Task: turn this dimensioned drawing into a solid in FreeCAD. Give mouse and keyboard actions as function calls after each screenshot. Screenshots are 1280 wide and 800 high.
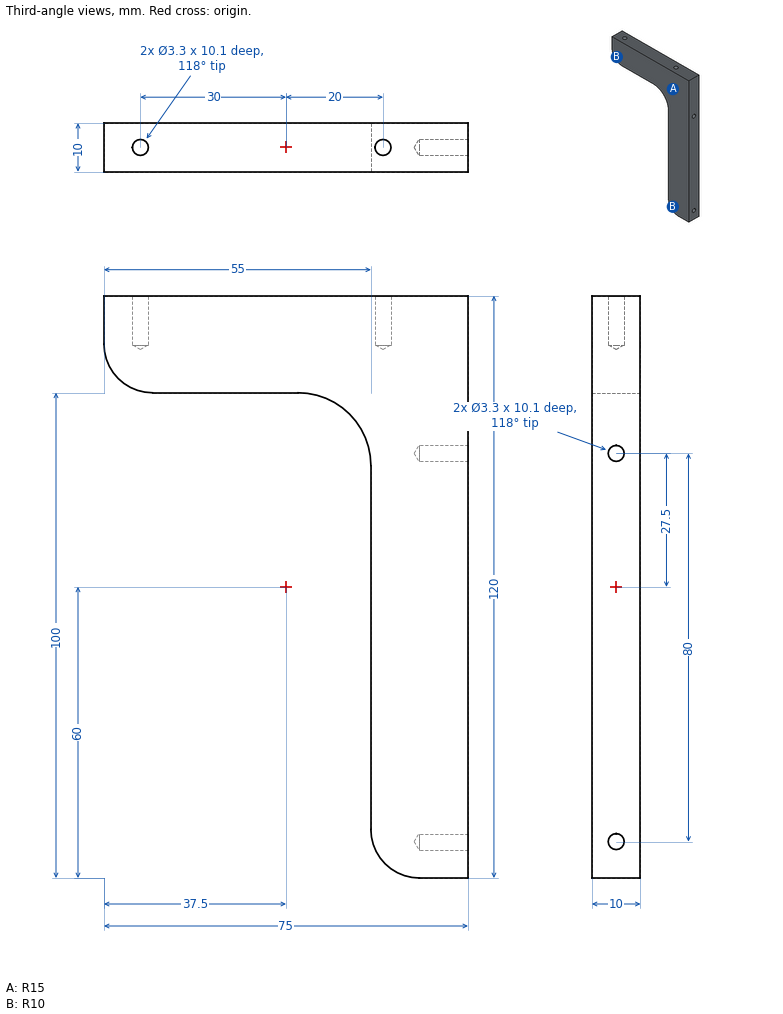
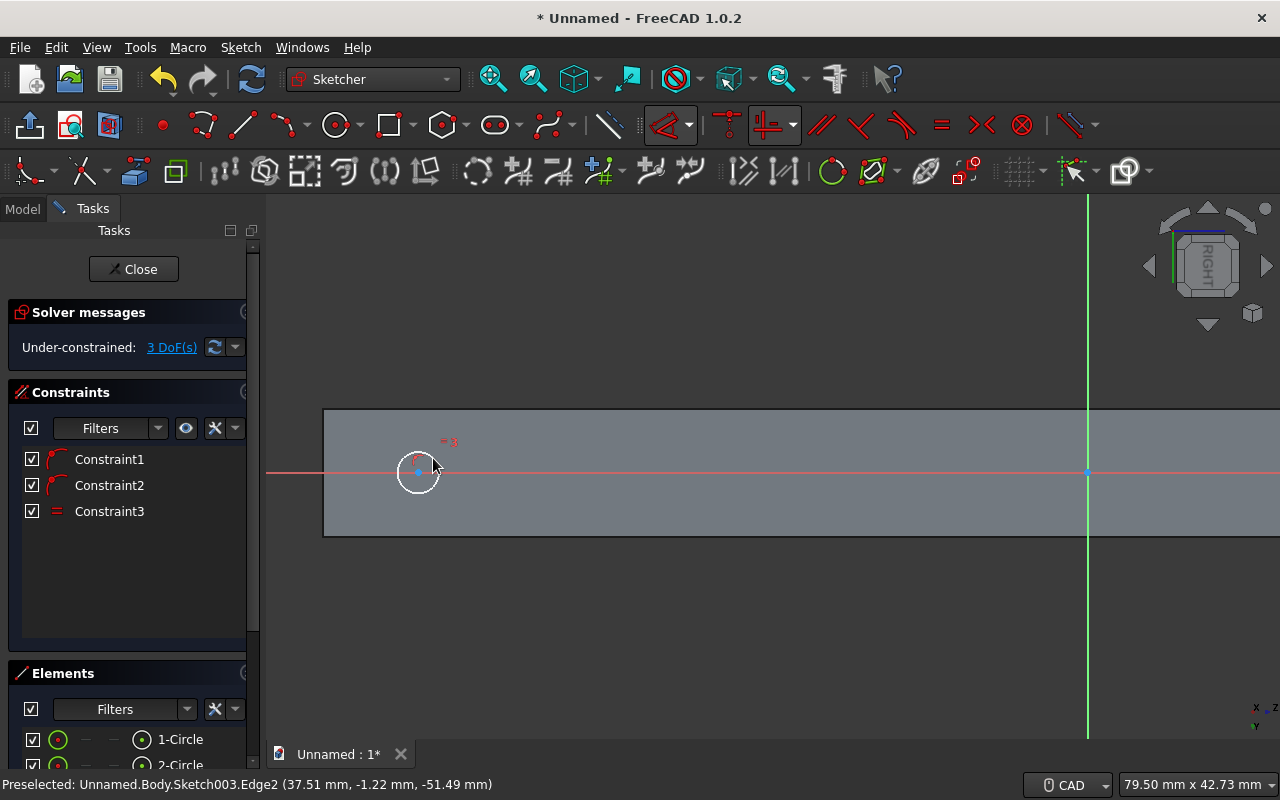
click(664, 126)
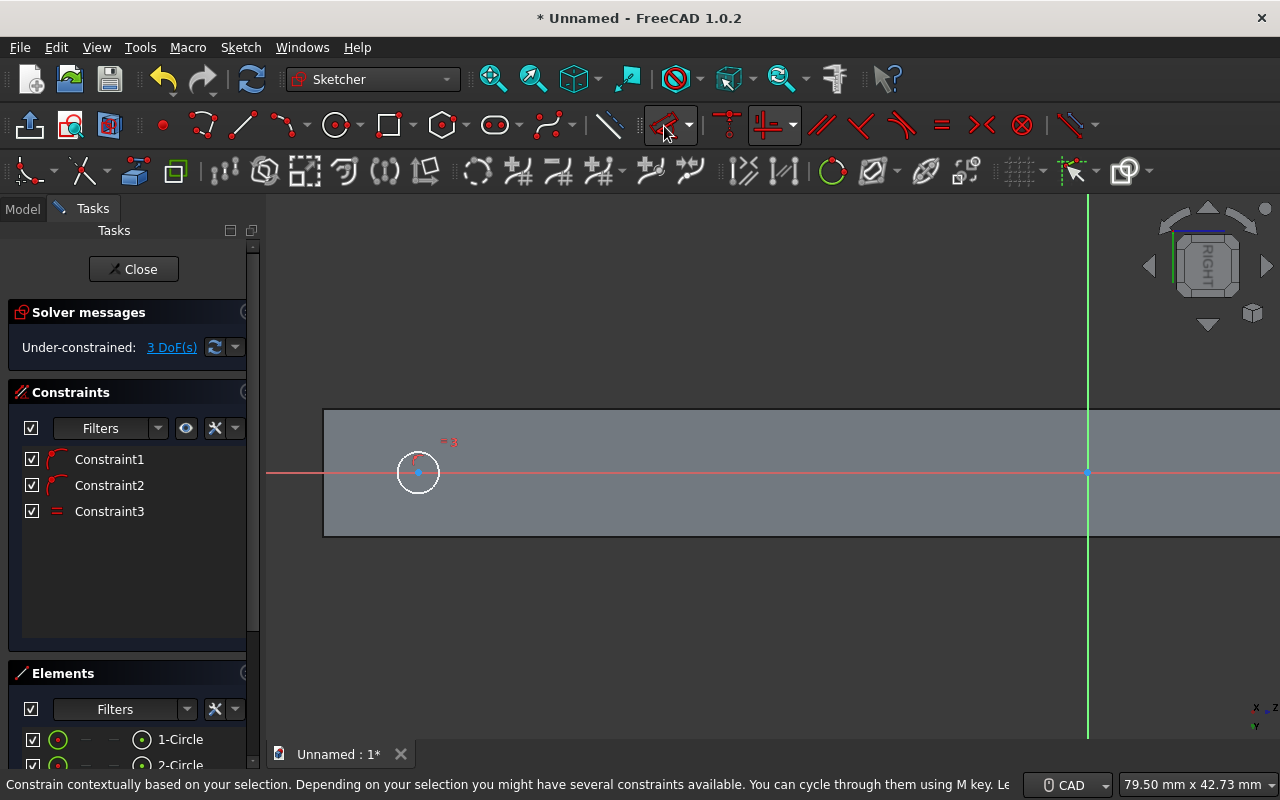
scroll(432, 459, down, 3)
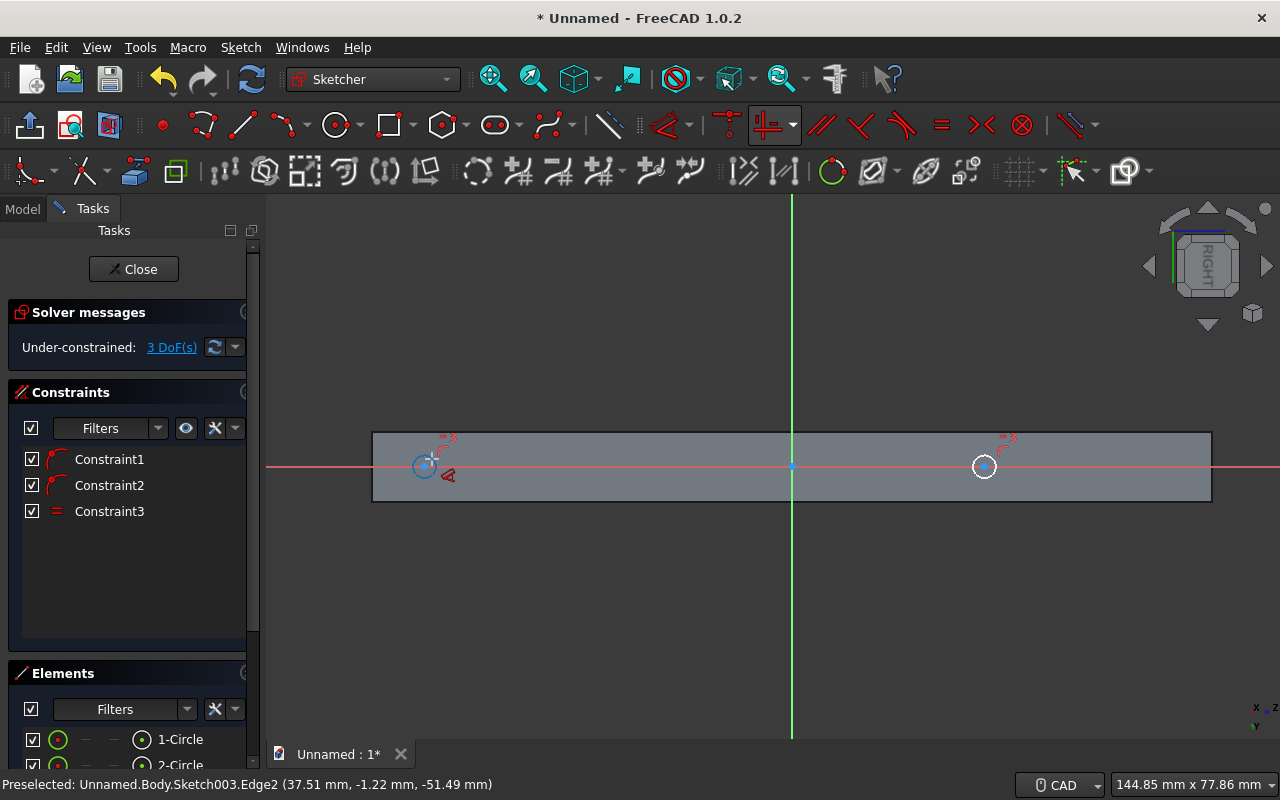
scroll(992, 459, up, 3)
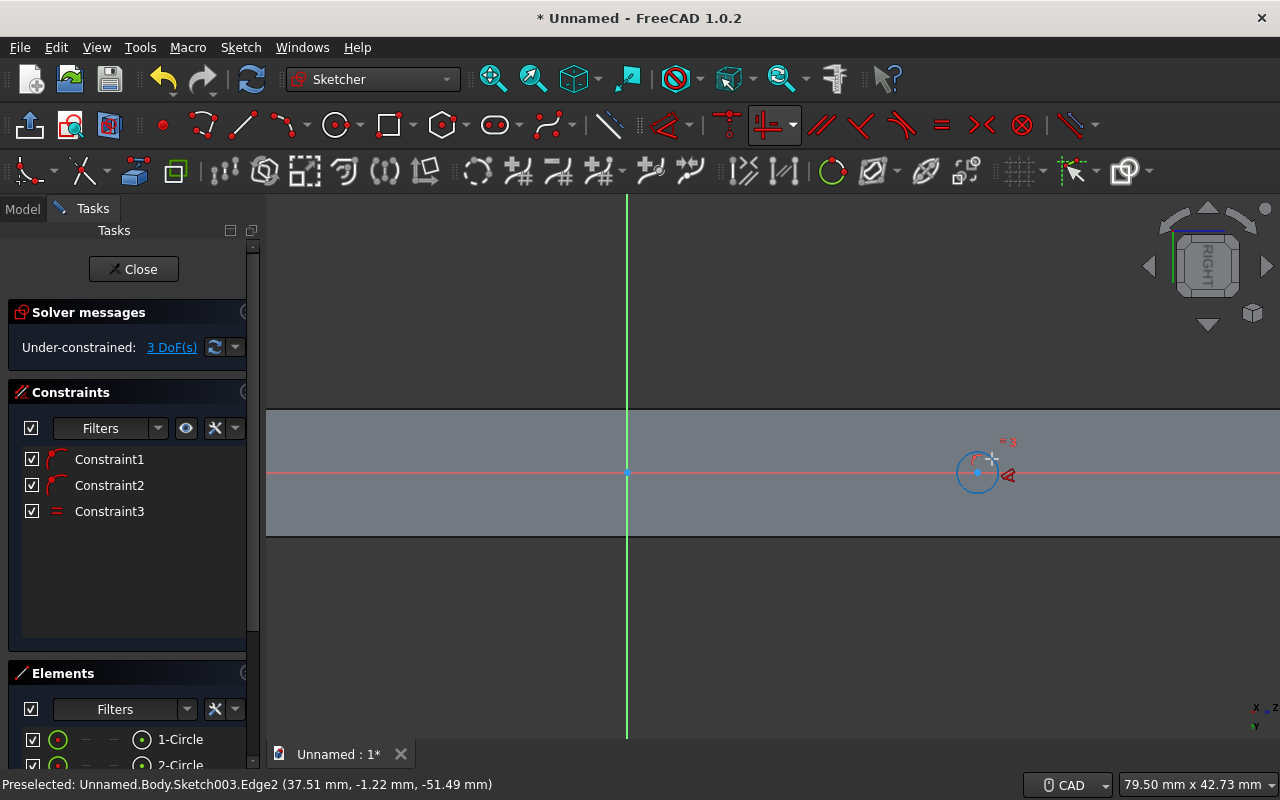
click(992, 458)
click(1014, 435)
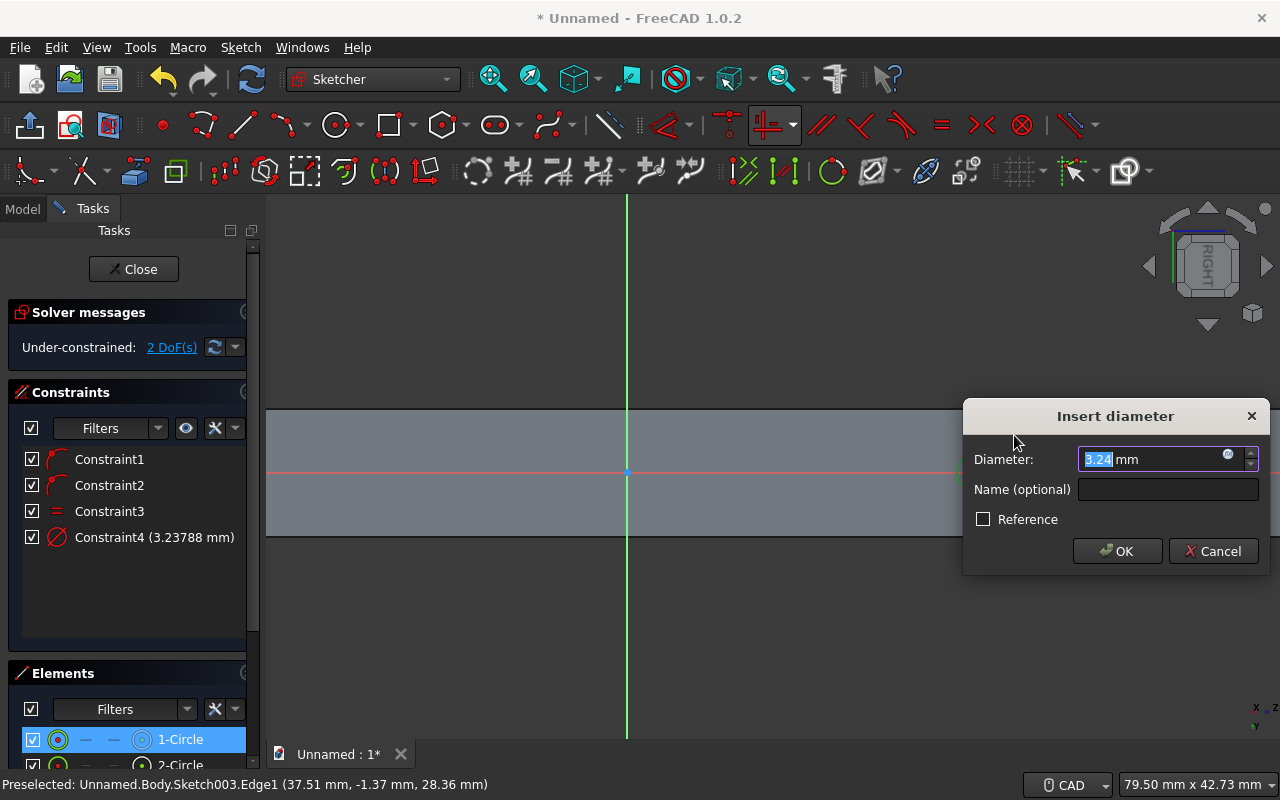
text(3.3)
key(Return)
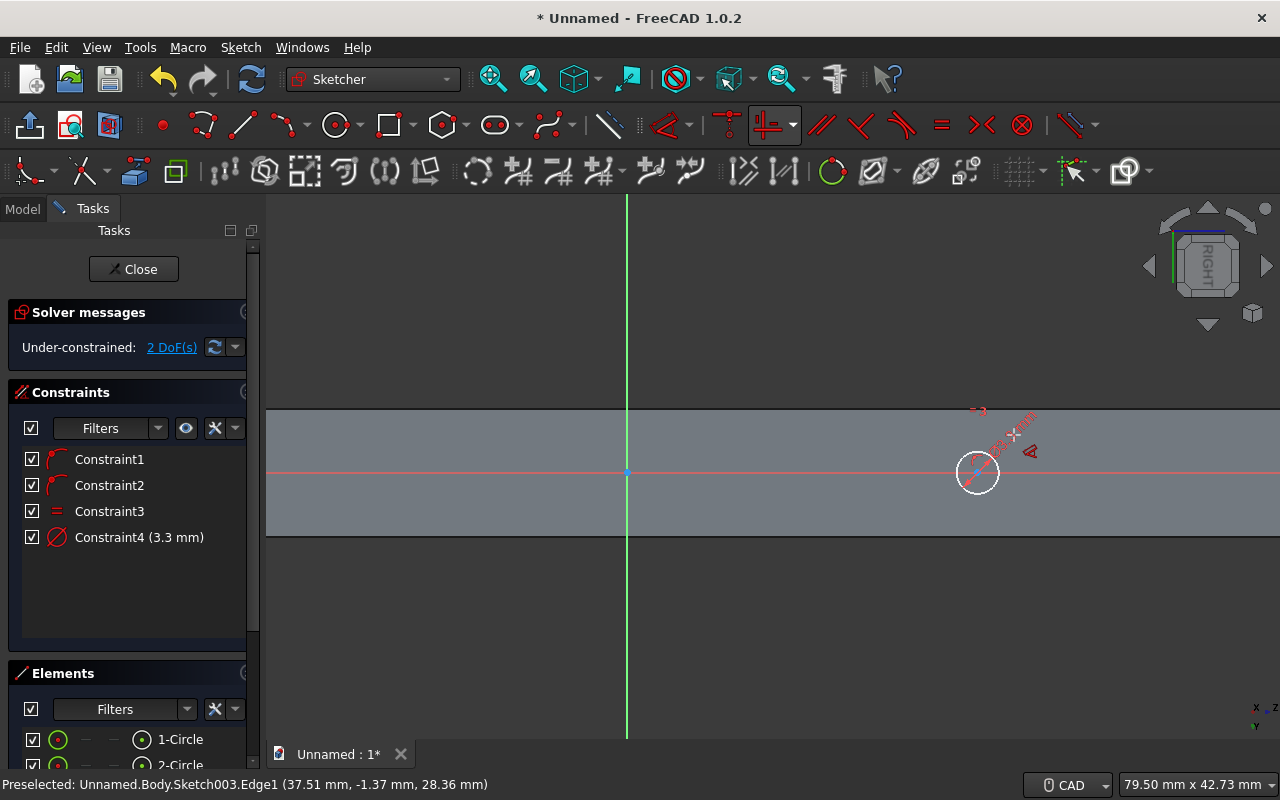
click(978, 473)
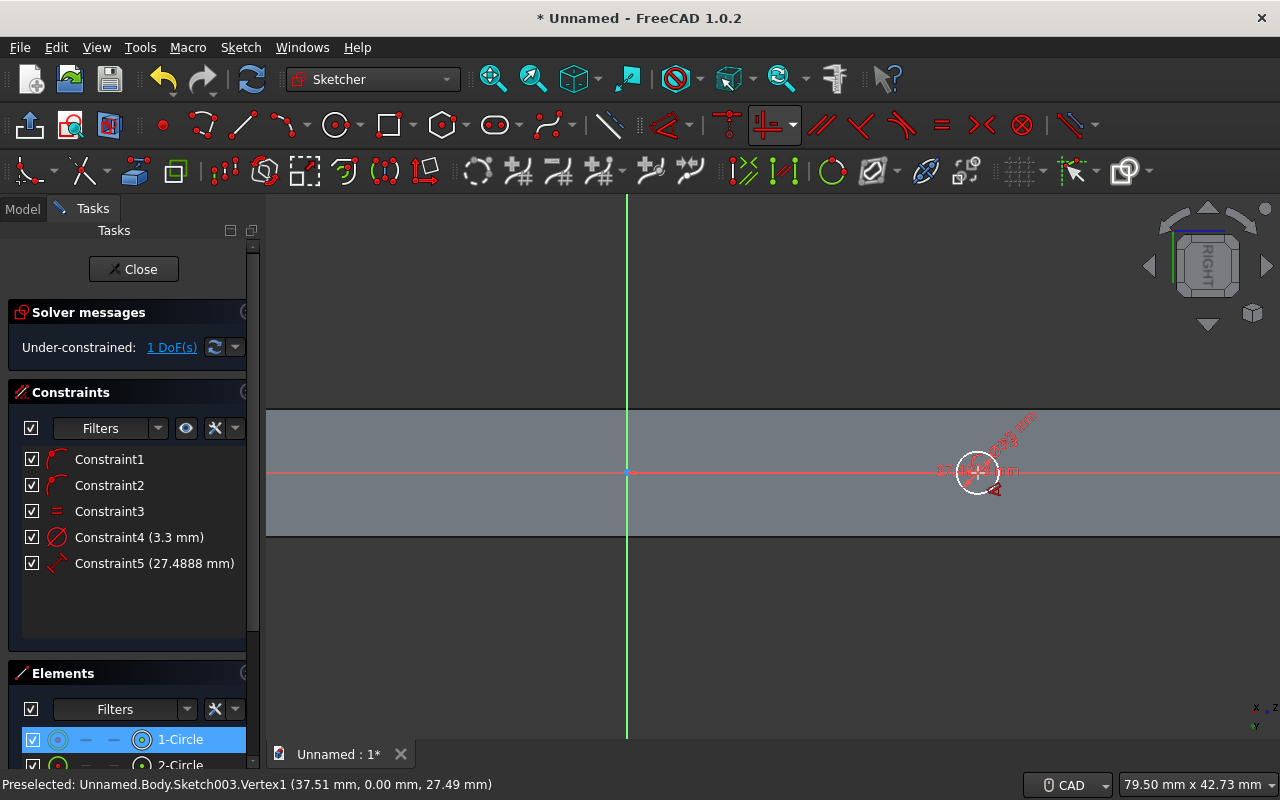
scroll(993, 459, down, 3)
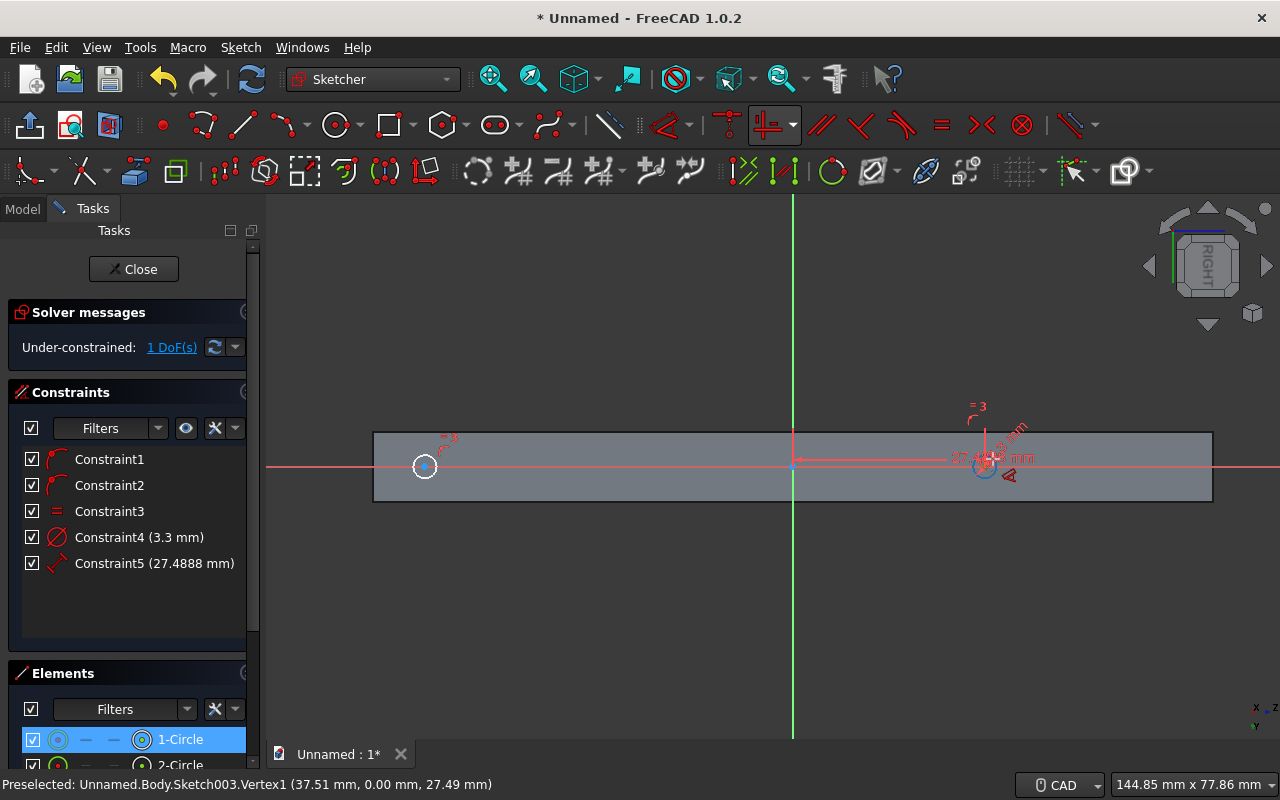
click(425, 467)
click(705, 501)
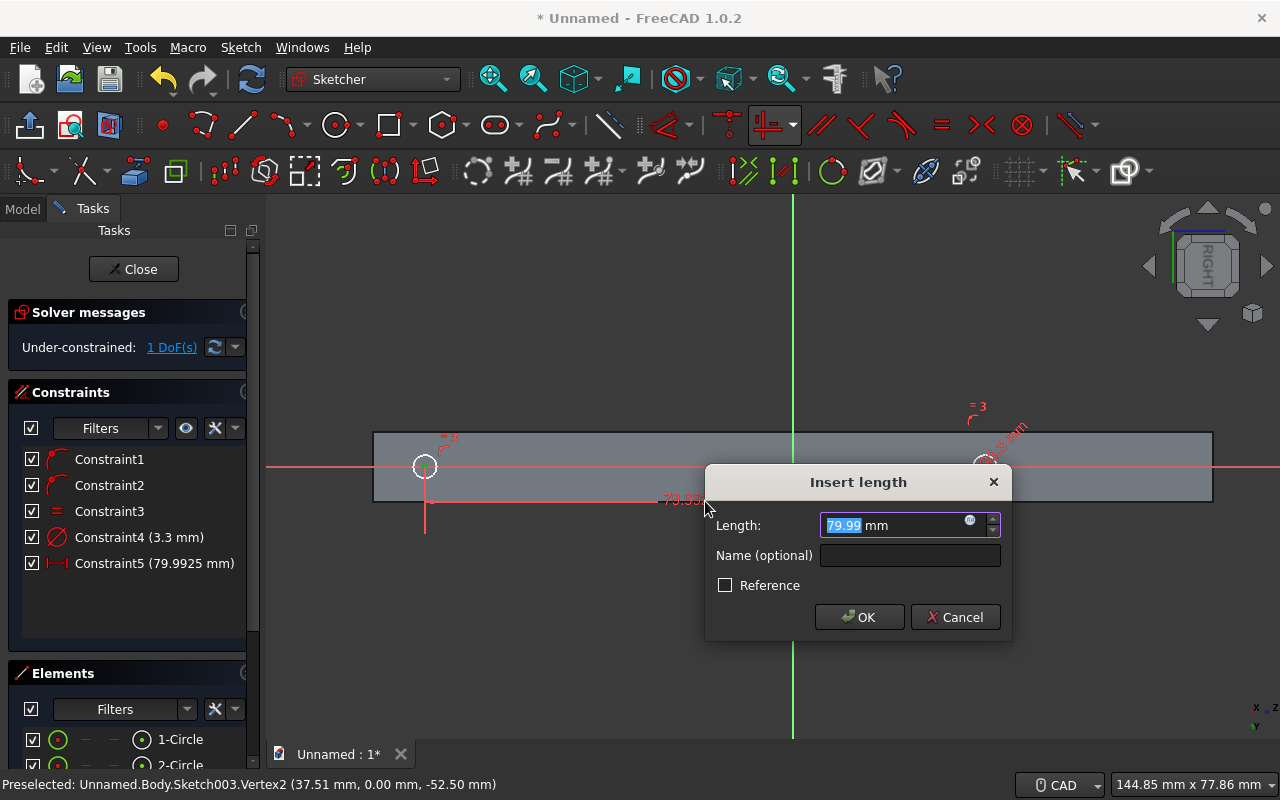
text(80)
key(Return)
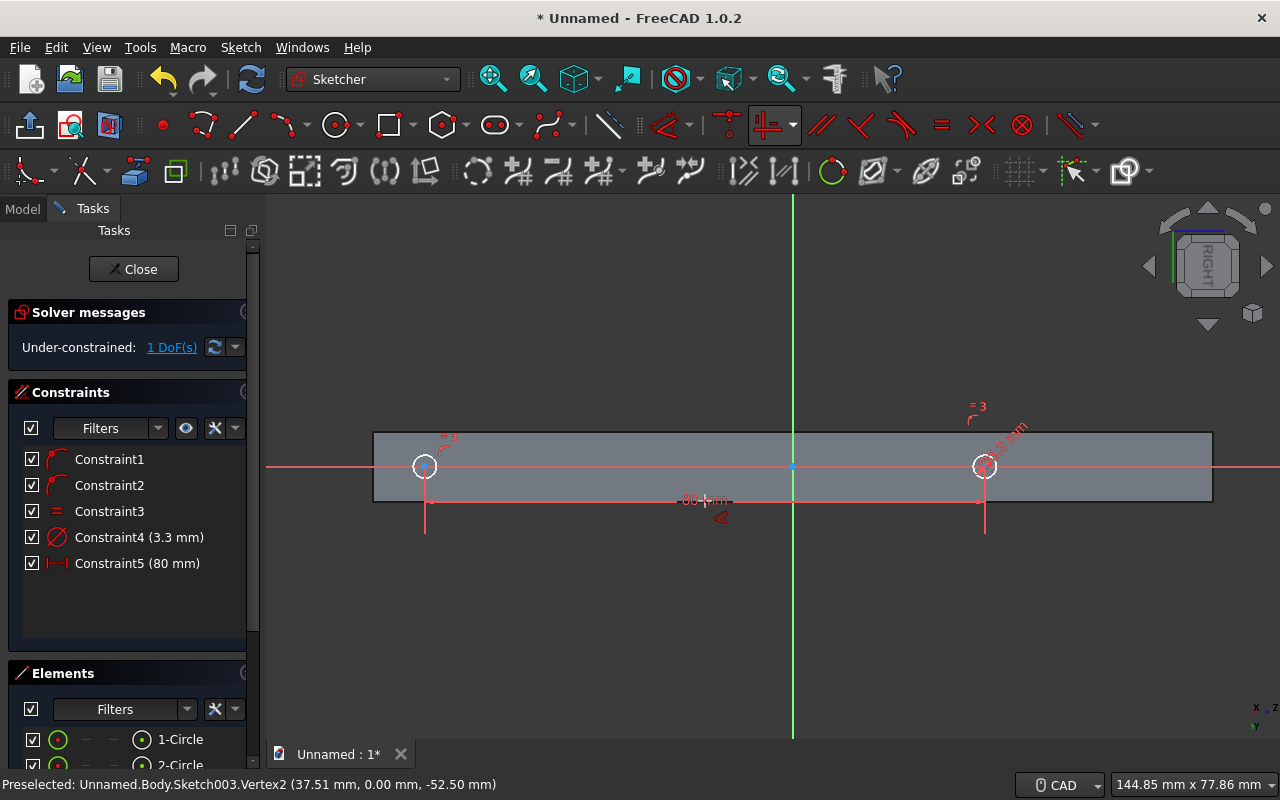
click(985, 467)
click(889, 501)